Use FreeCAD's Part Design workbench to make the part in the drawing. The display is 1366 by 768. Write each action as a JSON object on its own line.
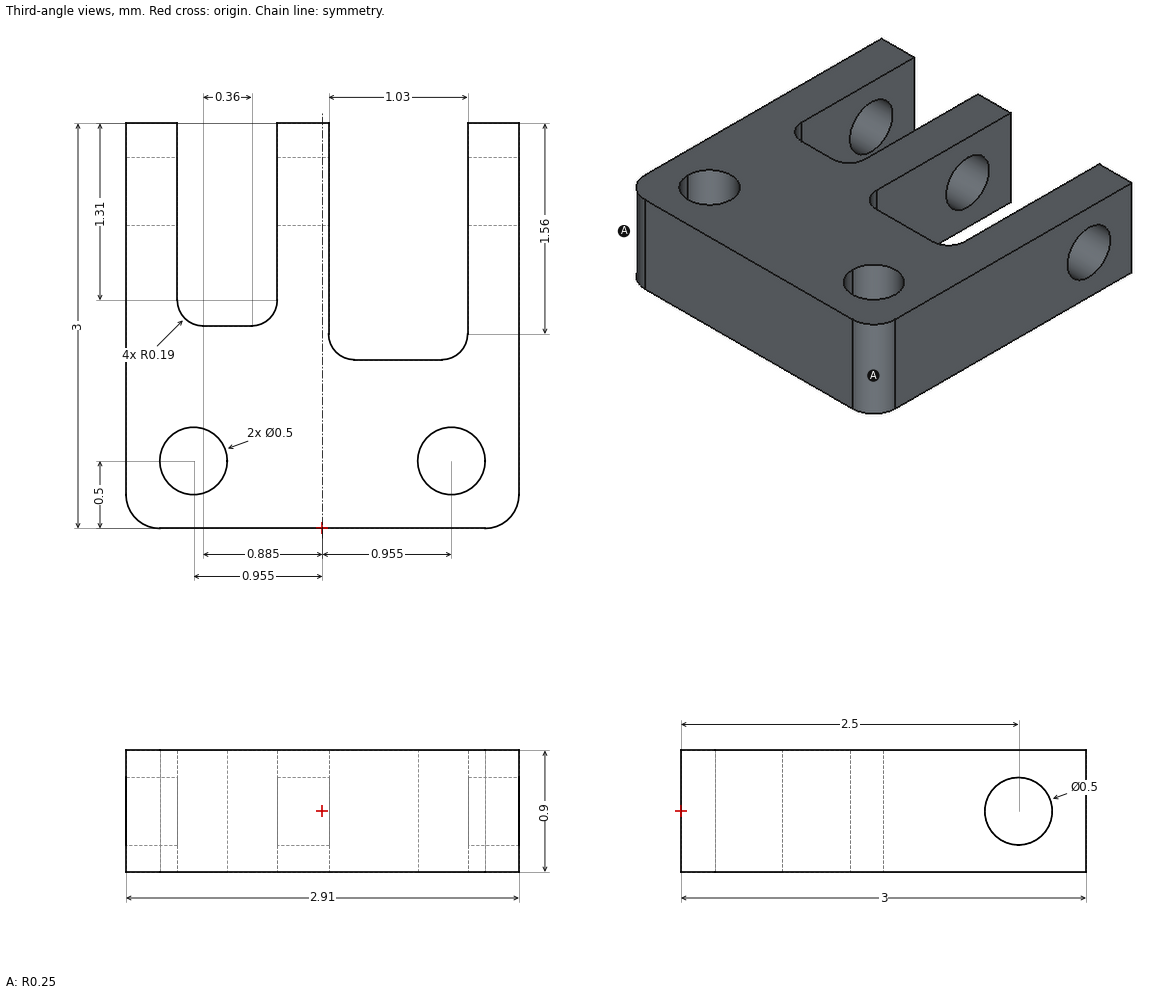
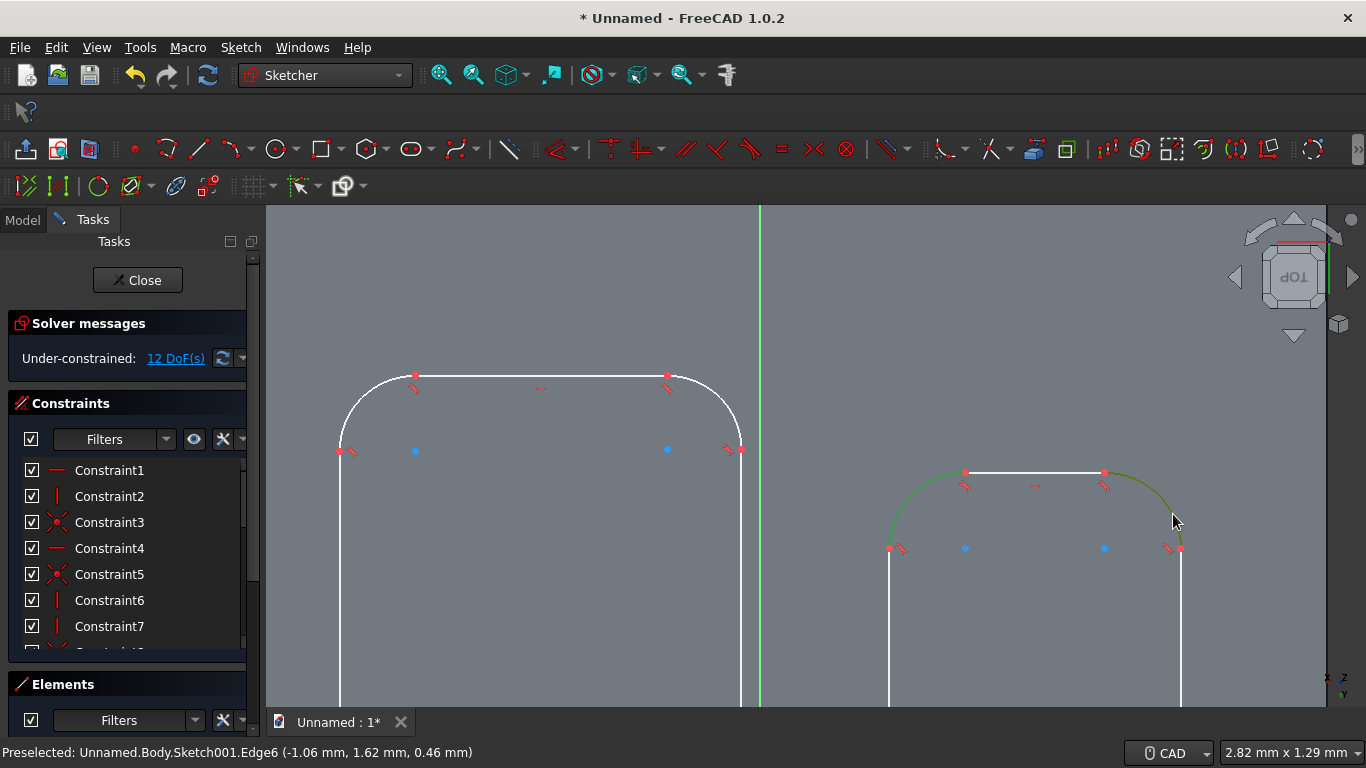
{"action": "left_click", "coordinate": [733, 416]}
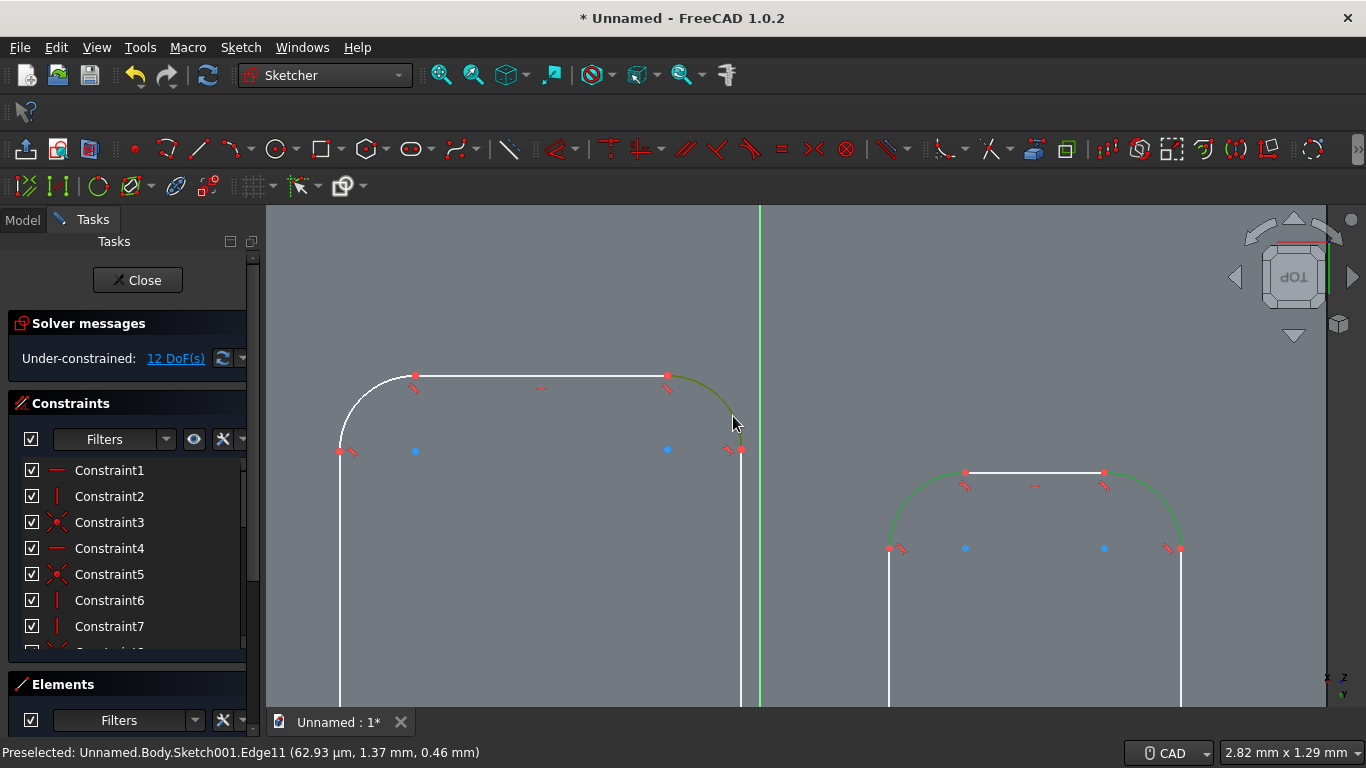
{"action": "left_click", "coordinate": [381, 384]}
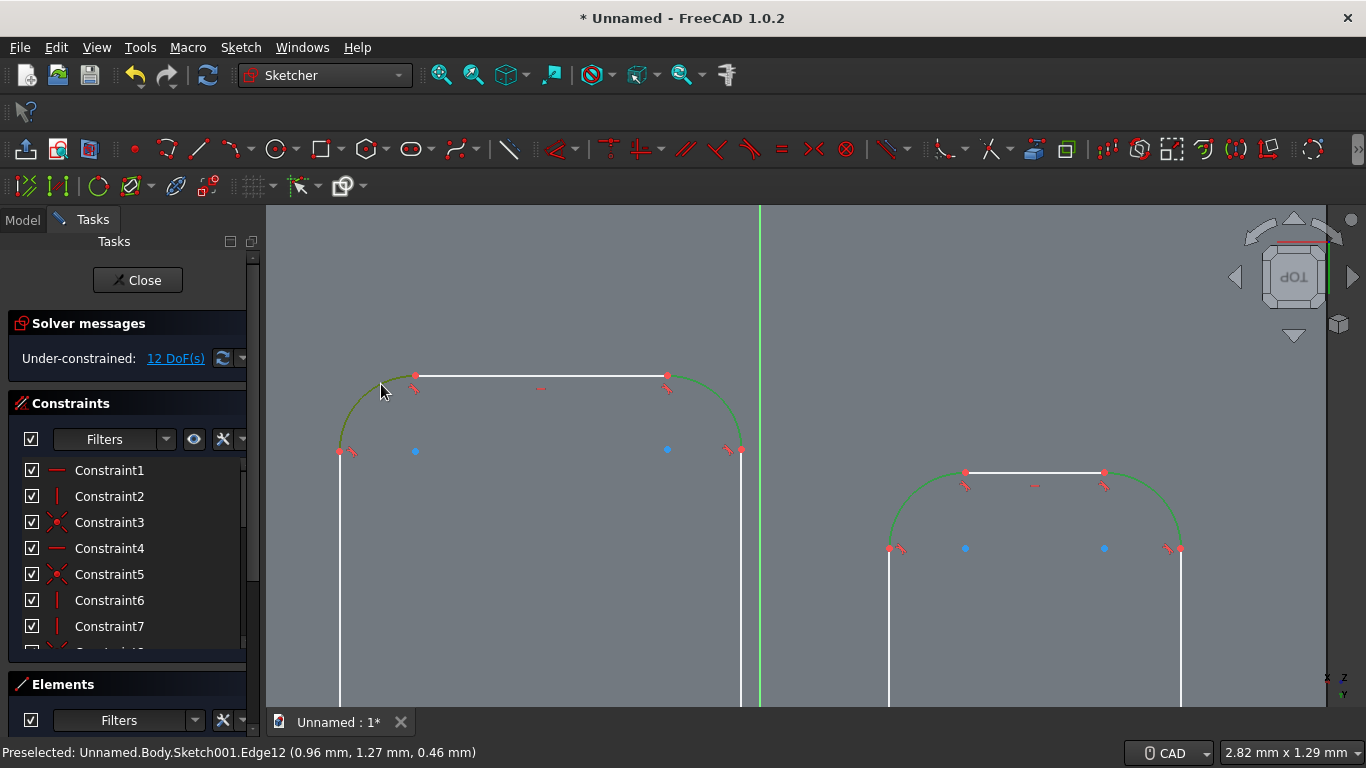
{"action": "key", "text": "e"}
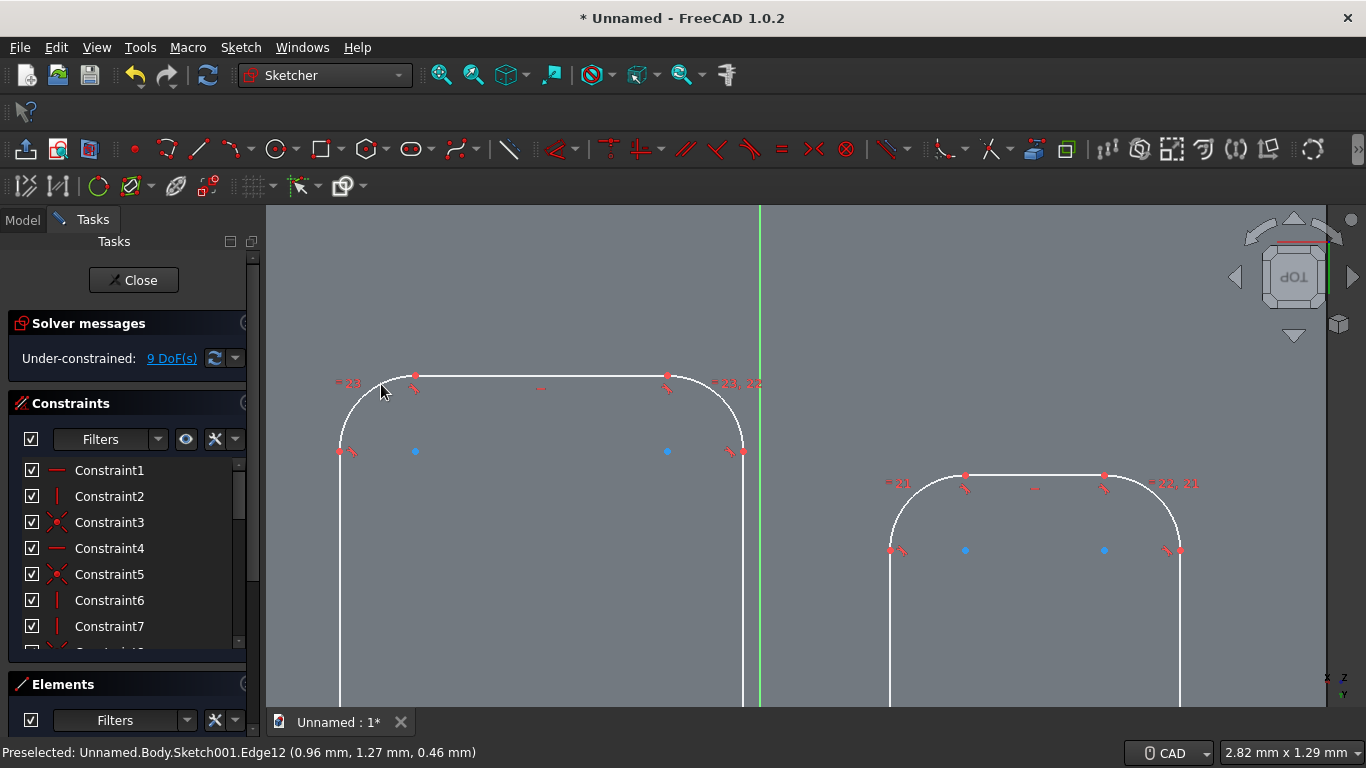
{"action": "scroll", "coordinate": [743, 451], "scroll_direction": "down", "scroll_amount": 7}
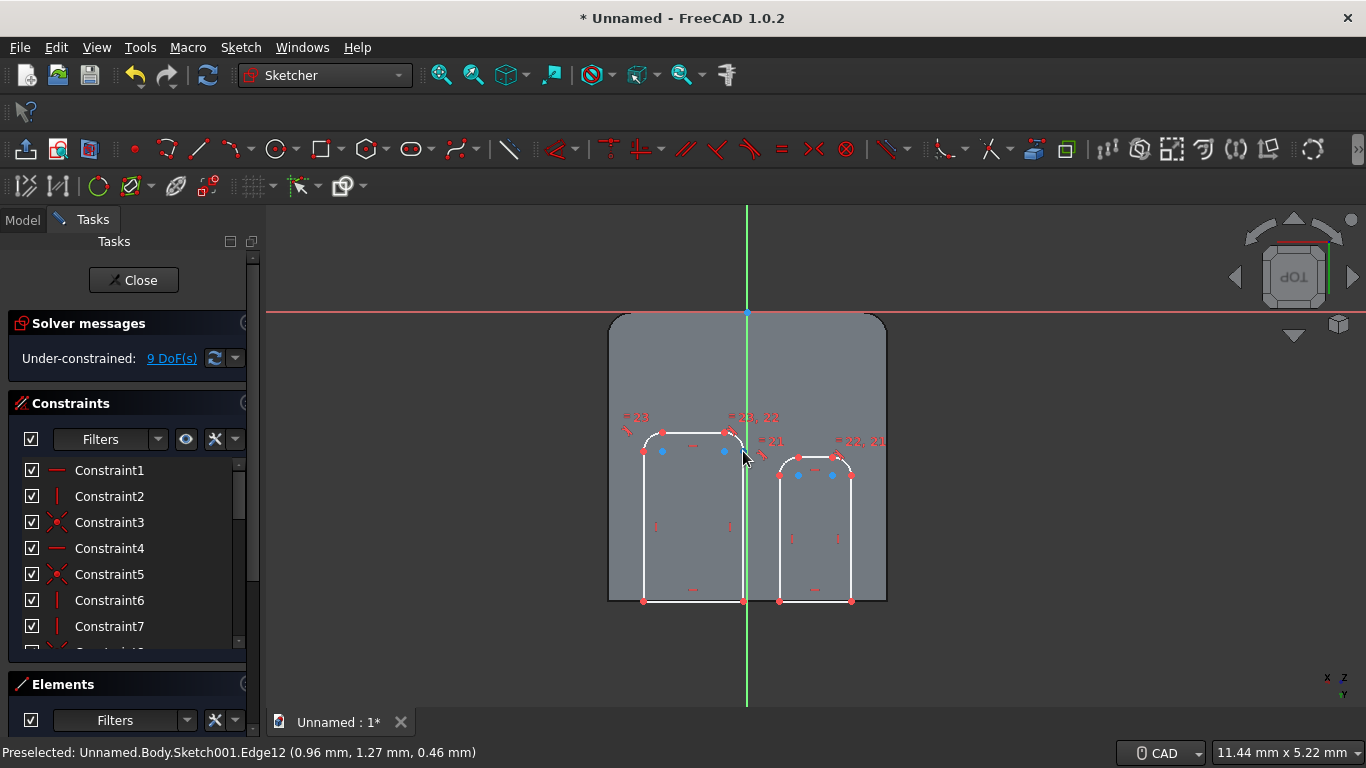
{"action": "left_click", "coordinate": [851, 602]}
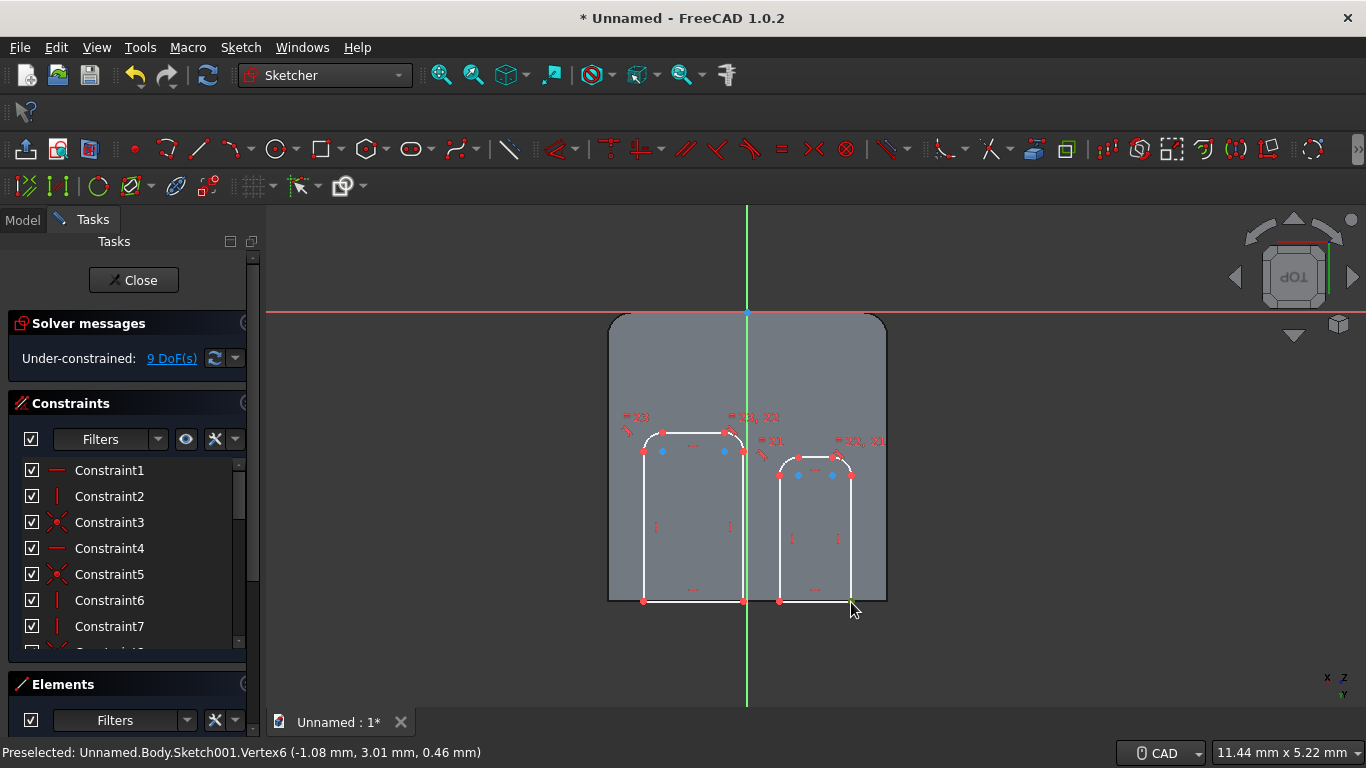
{"action": "left_click", "coordinate": [644, 602]}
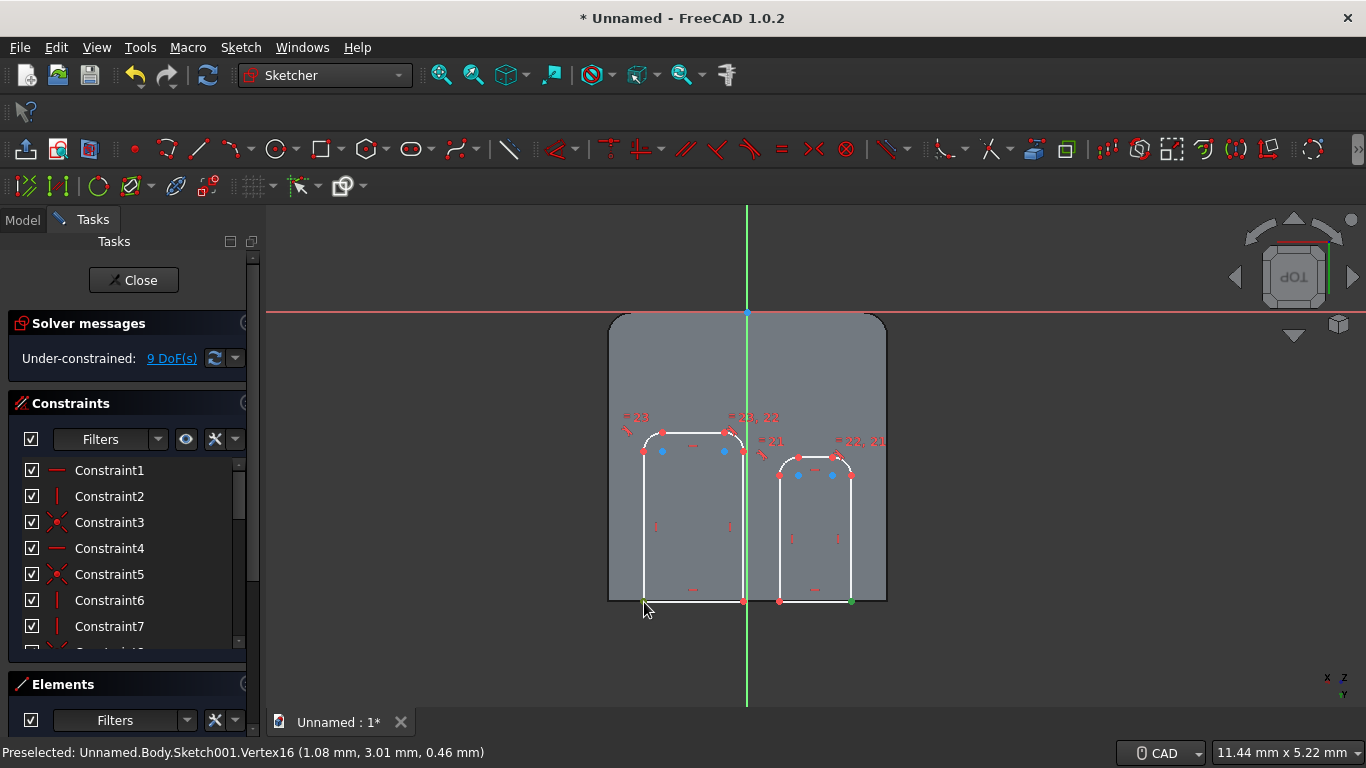
{"action": "left_click", "coordinate": [747, 647]}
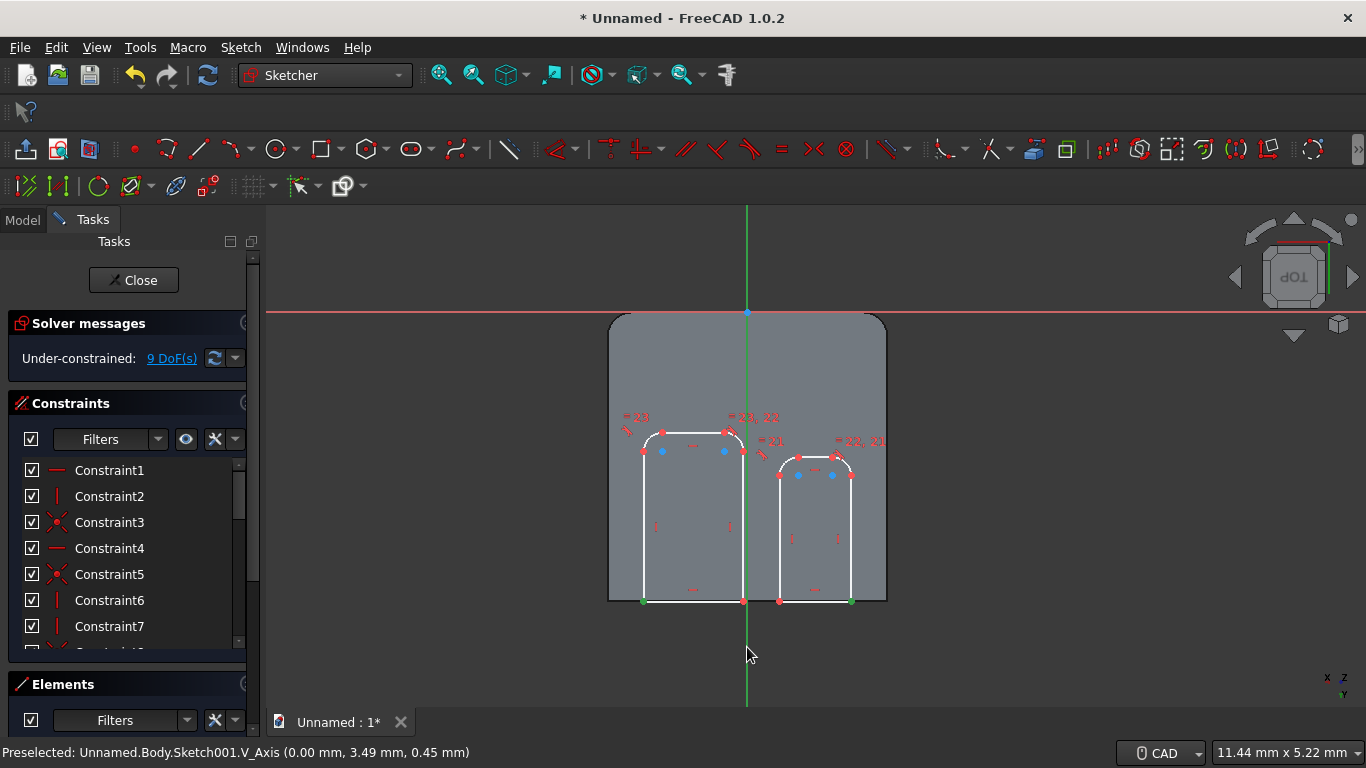
{"action": "left_click", "coordinate": [814, 150]}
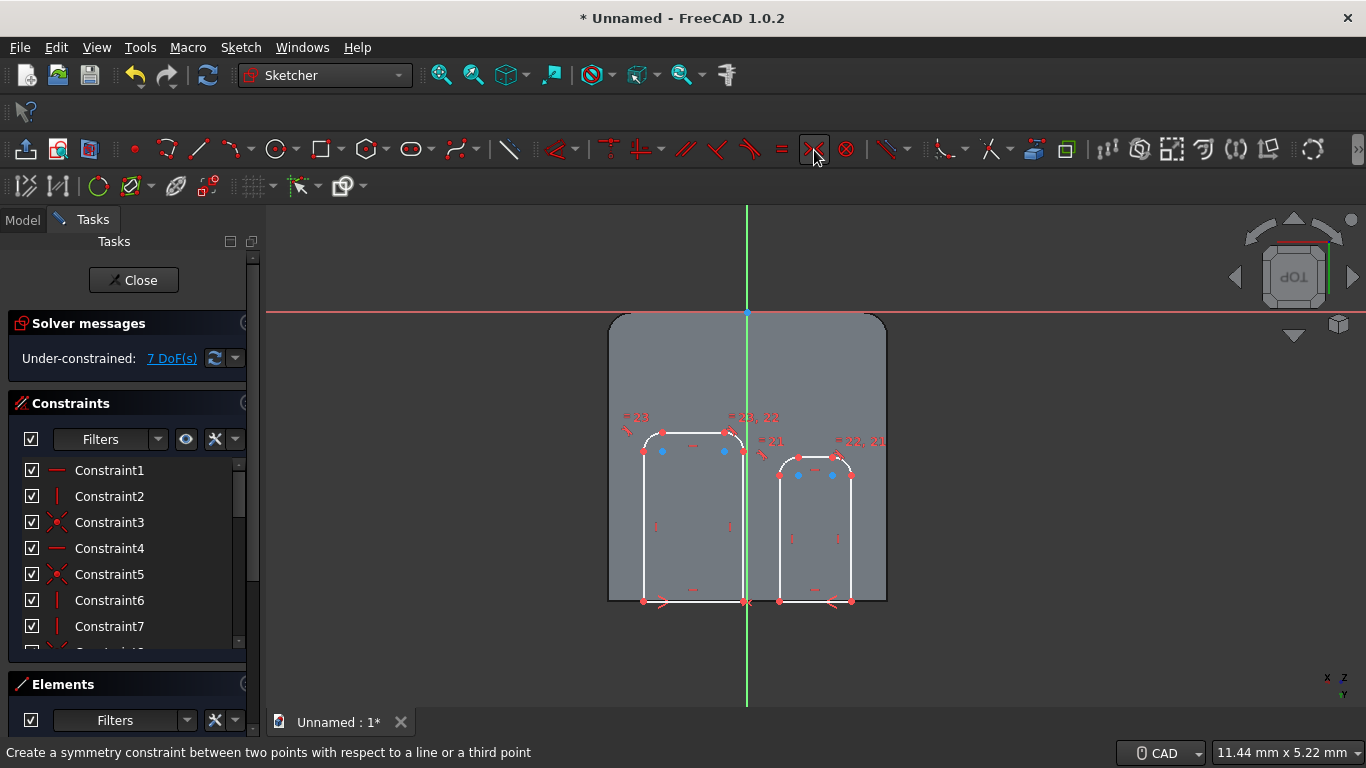
{"action": "key", "text": "d"}